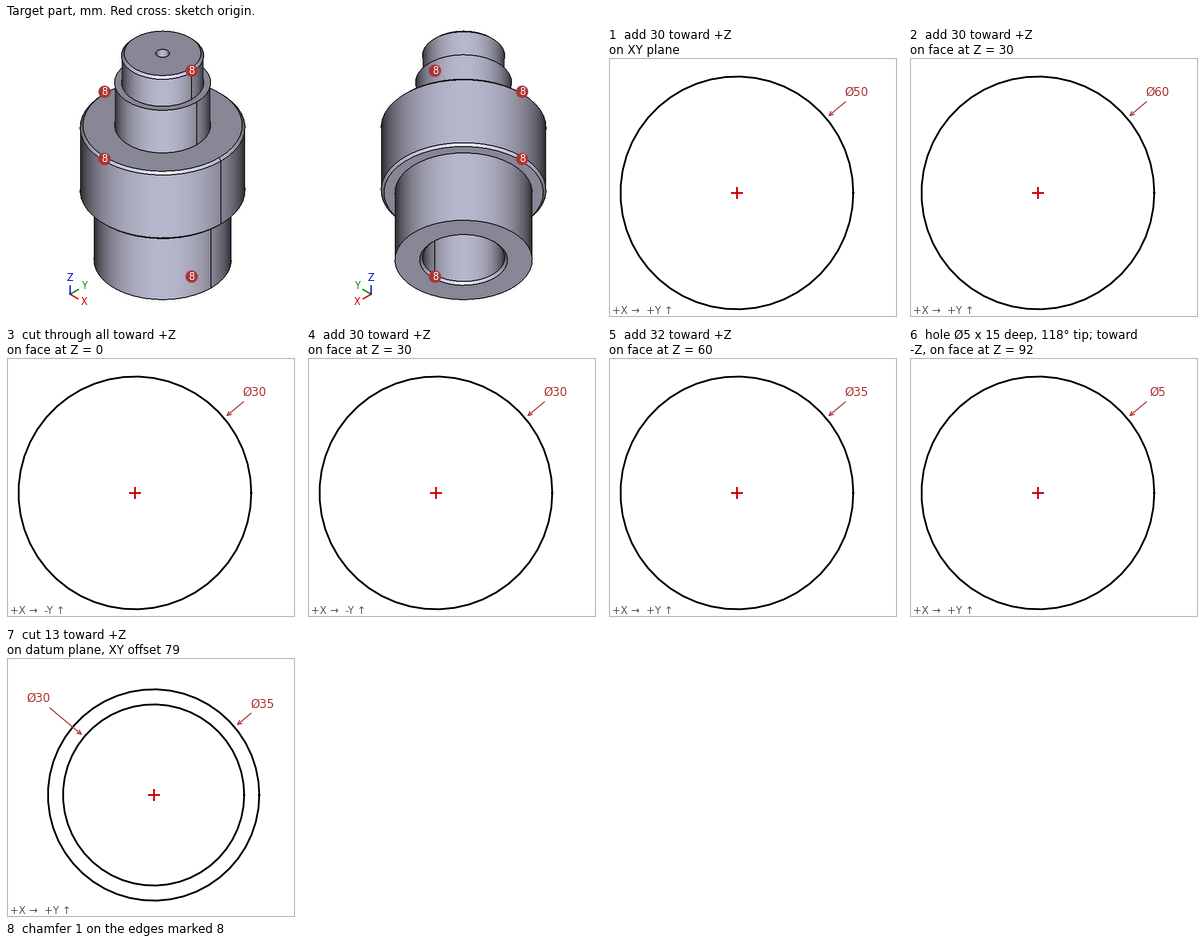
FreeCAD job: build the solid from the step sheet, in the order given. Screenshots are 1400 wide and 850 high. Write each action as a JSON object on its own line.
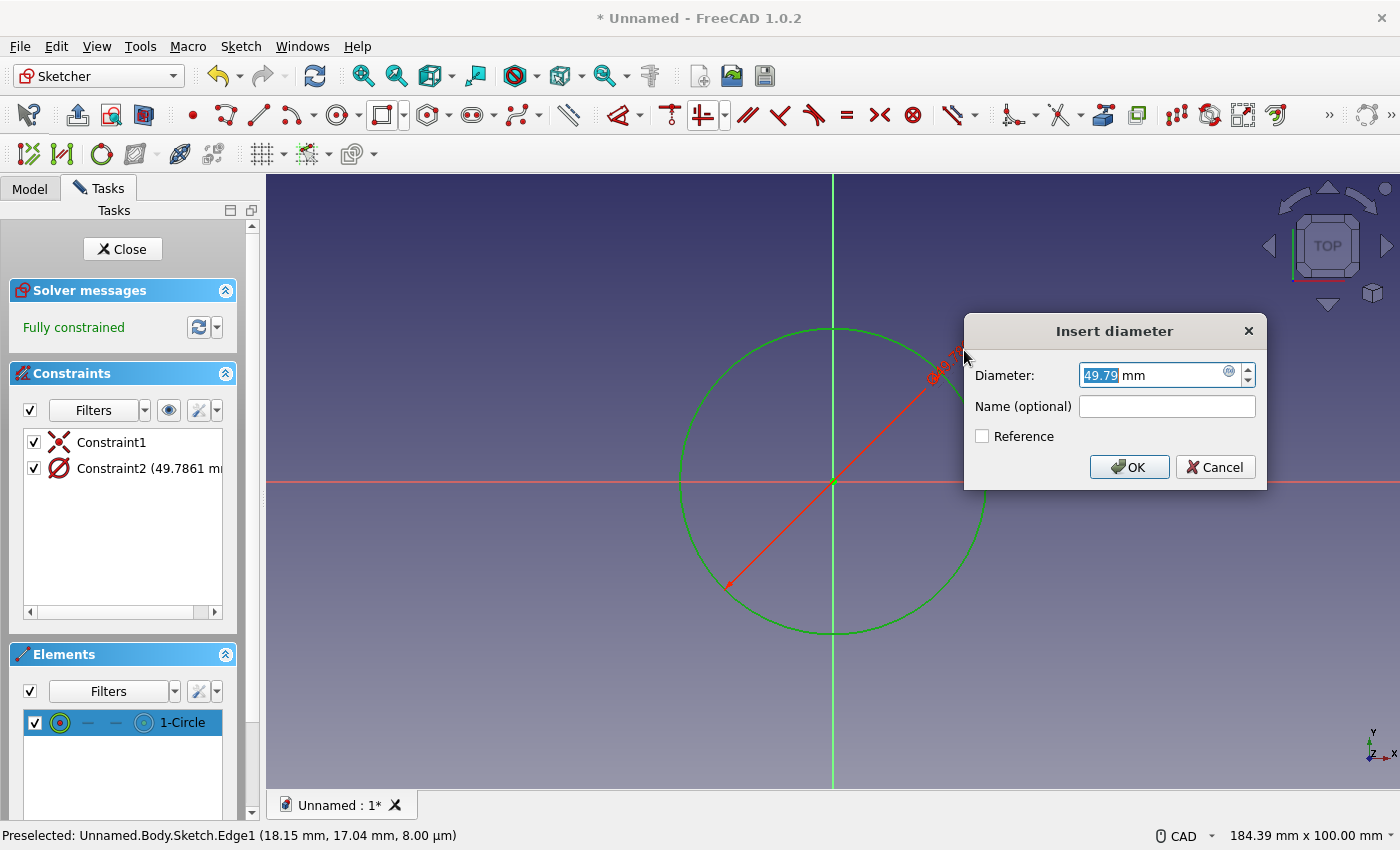
{"action": "type", "text": "50"}
{"action": "key", "text": "Return"}
{"action": "key", "text": "Escape"}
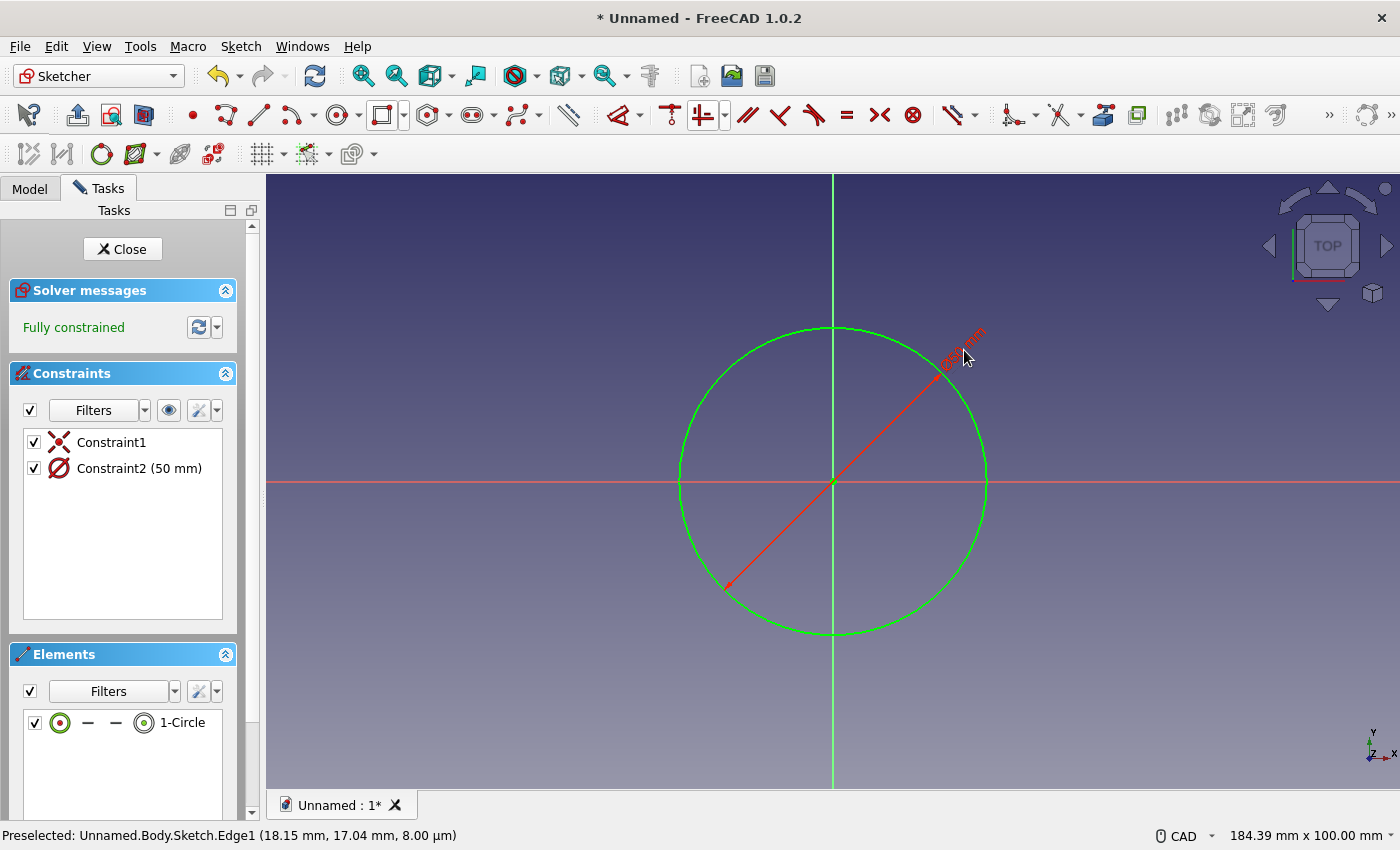
{"action": "left_click", "coordinate": [123, 249]}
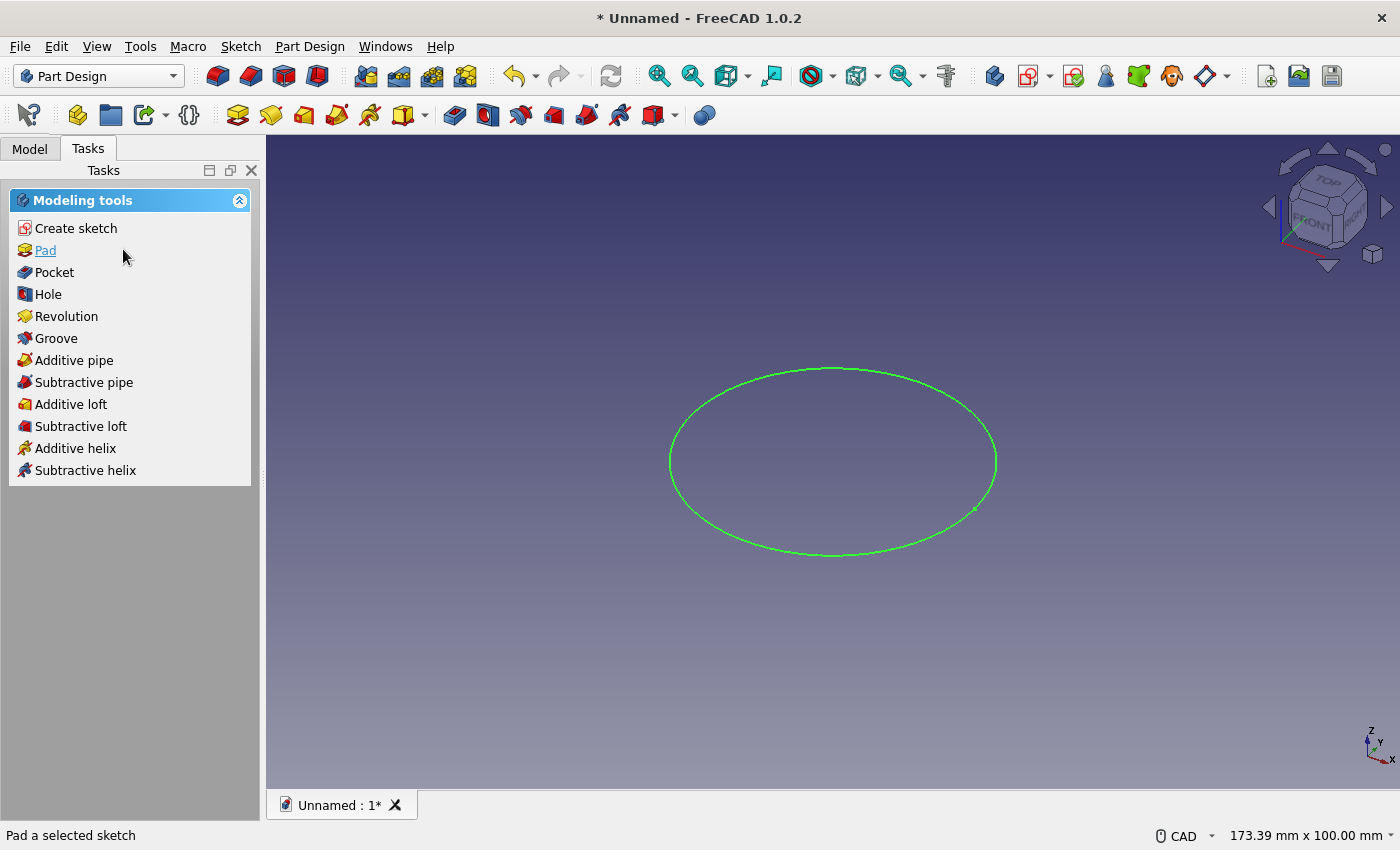
{"action": "left_click", "coordinate": [238, 116]}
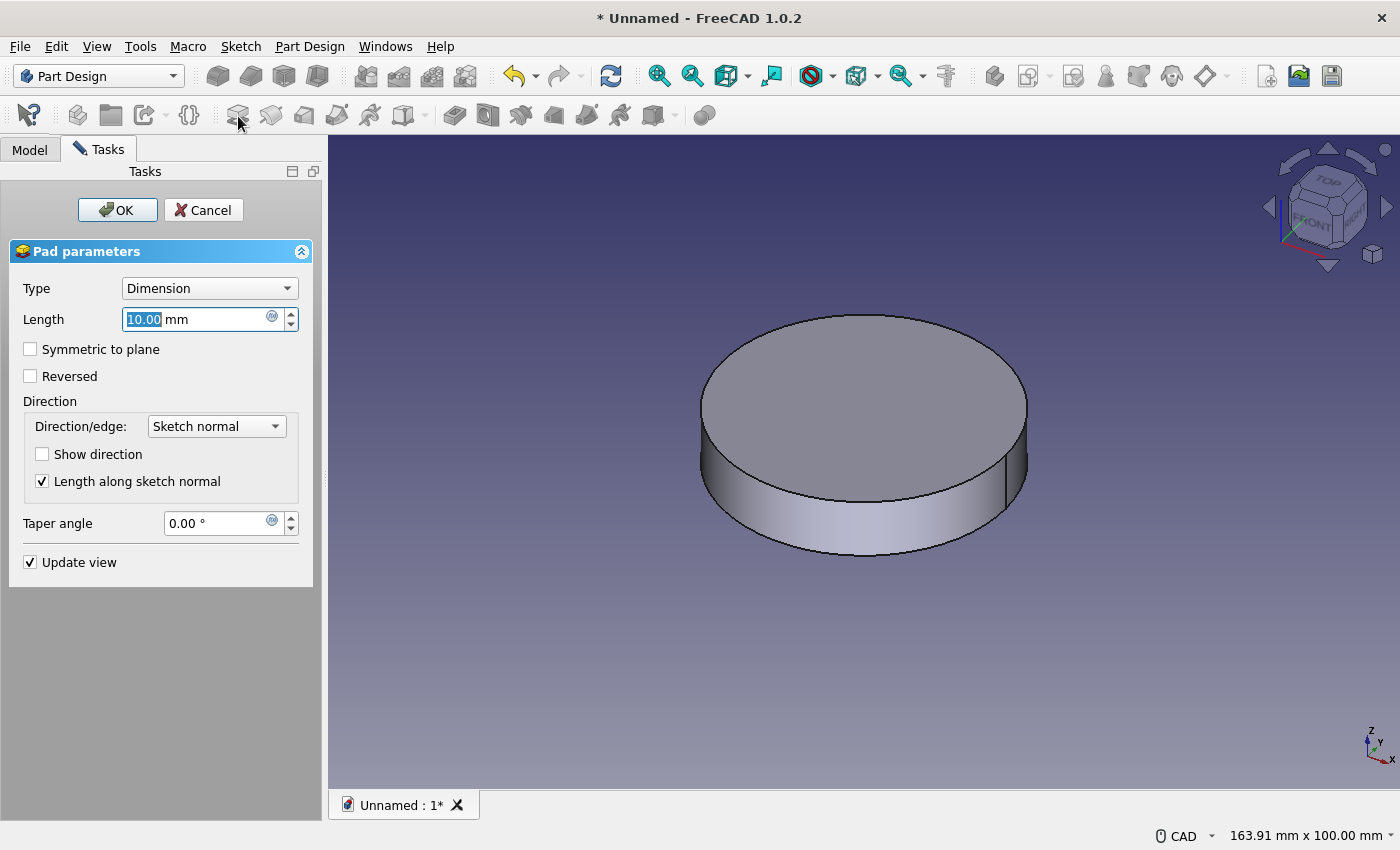
{"action": "type", "text": "30"}
{"action": "key", "text": "Tab"}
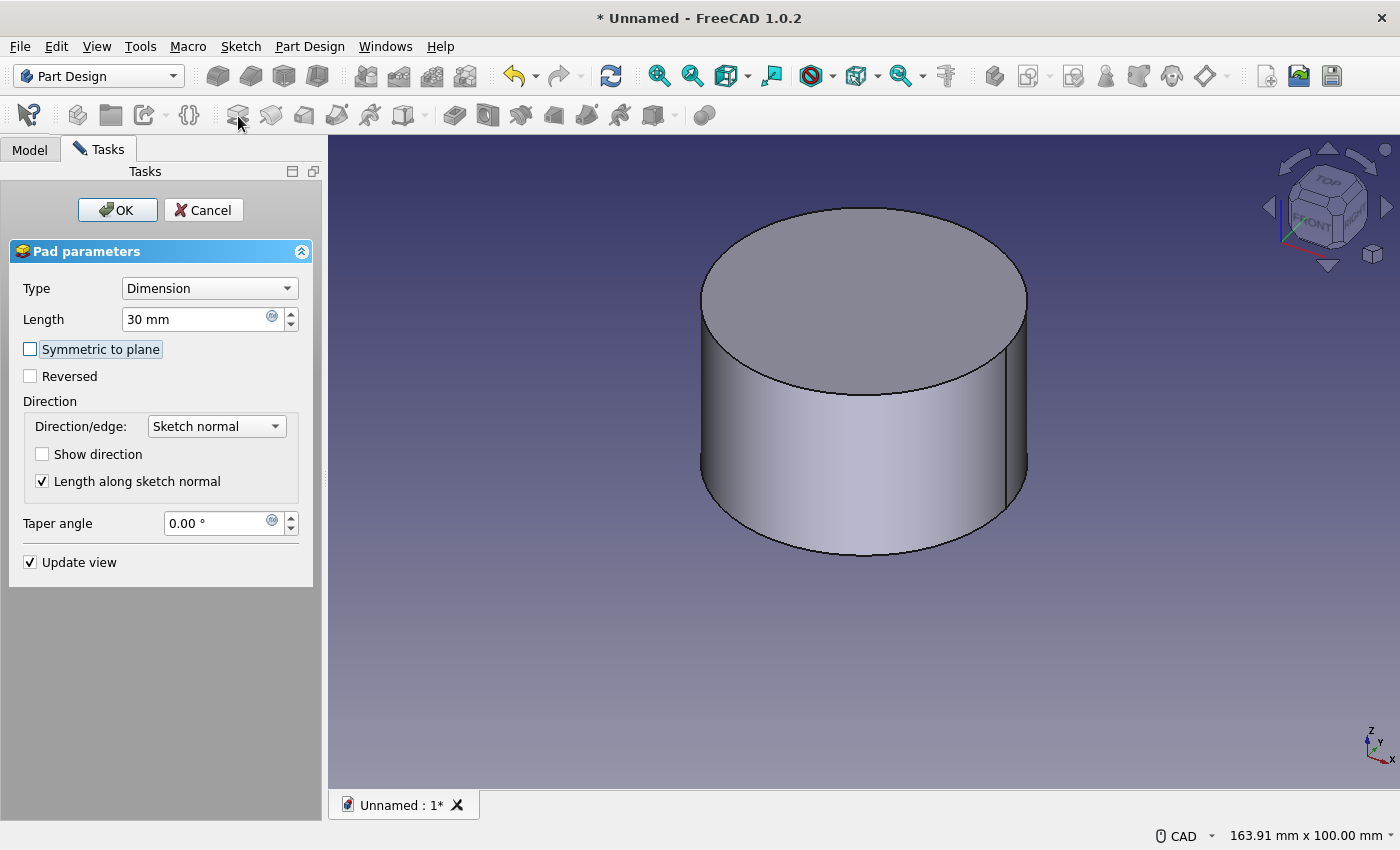
{"action": "left_click", "coordinate": [118, 210]}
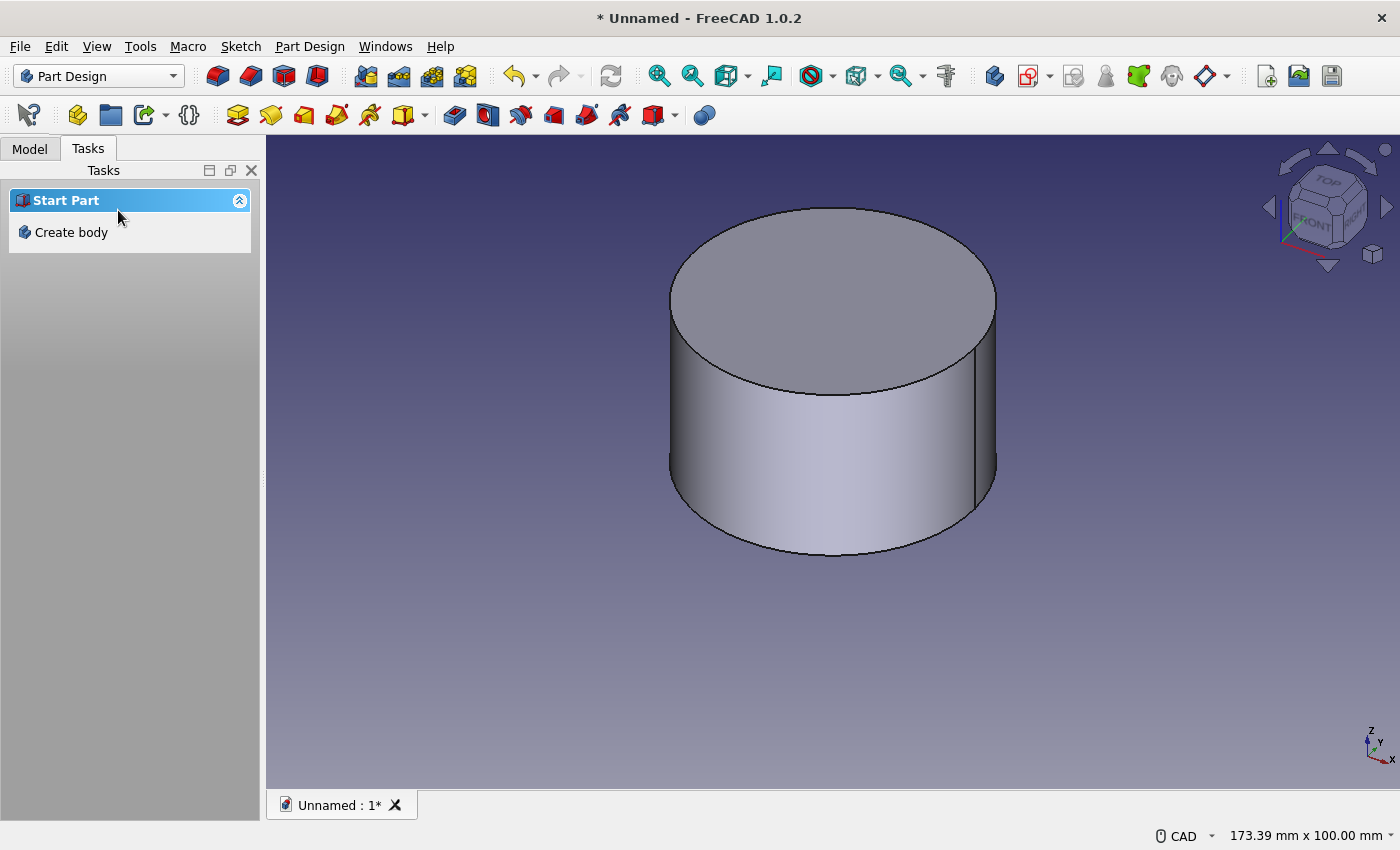
{"action": "left_click", "coordinate": [833, 300]}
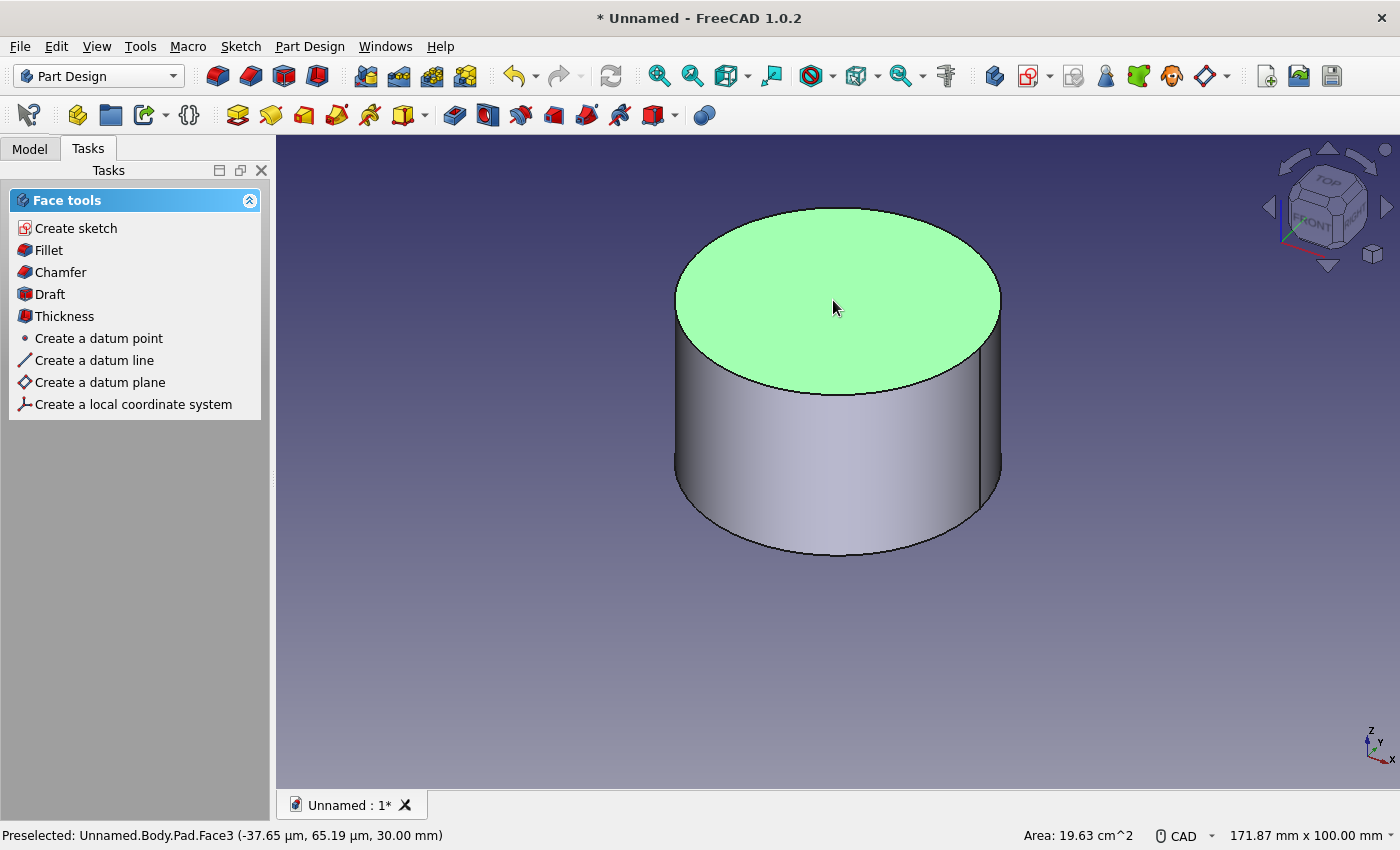
{"action": "left_click", "coordinate": [1028, 76]}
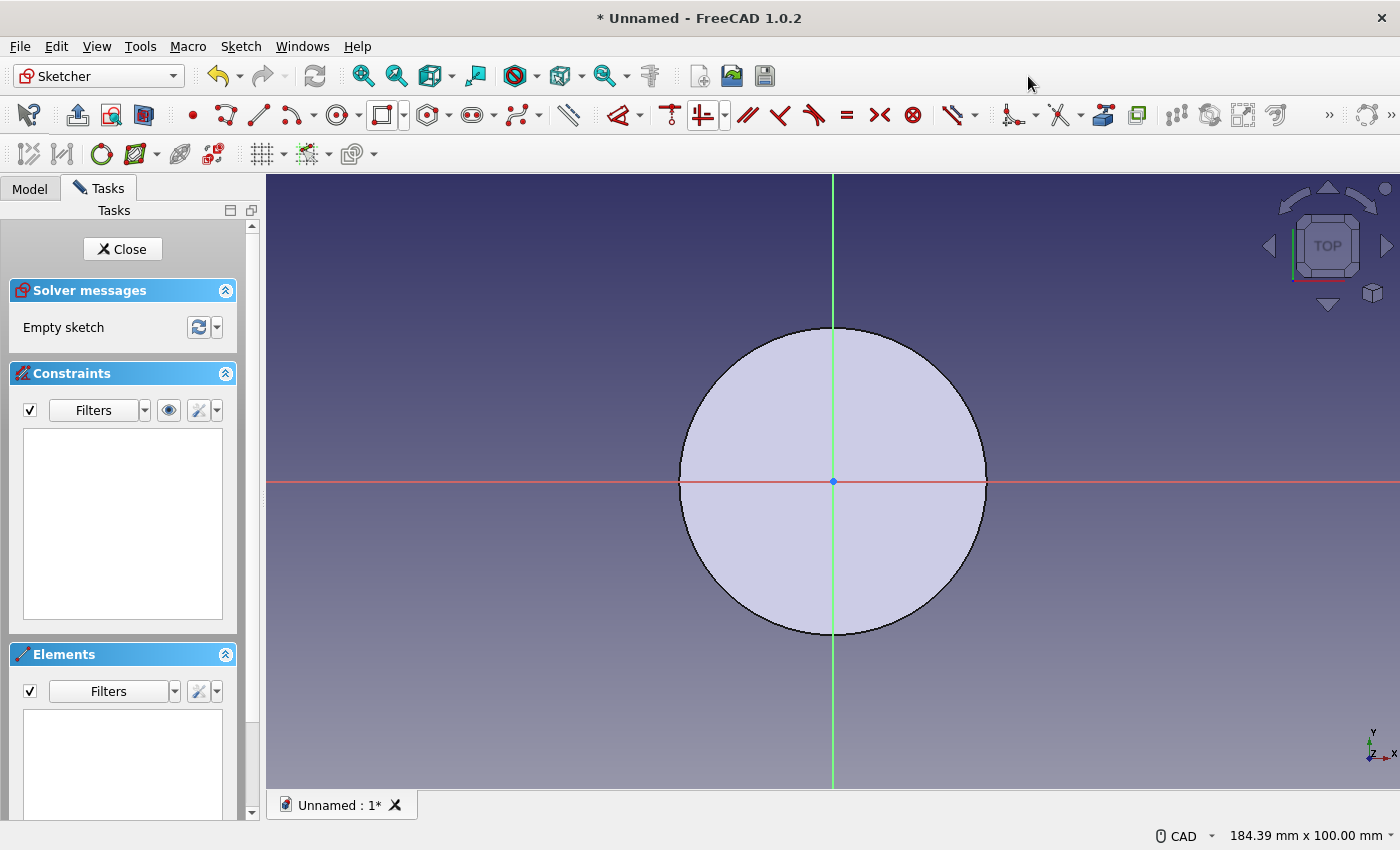
{"action": "left_click", "coordinate": [336, 116]}